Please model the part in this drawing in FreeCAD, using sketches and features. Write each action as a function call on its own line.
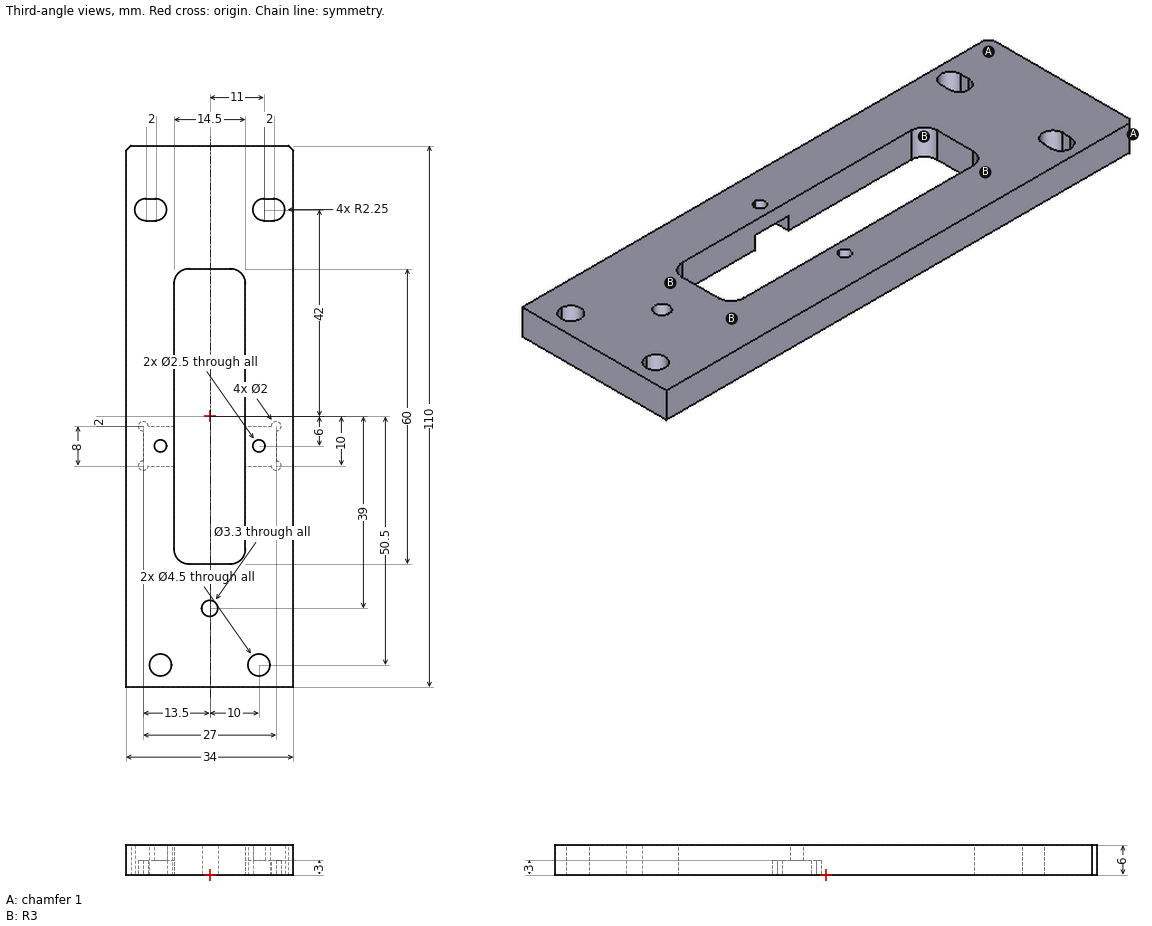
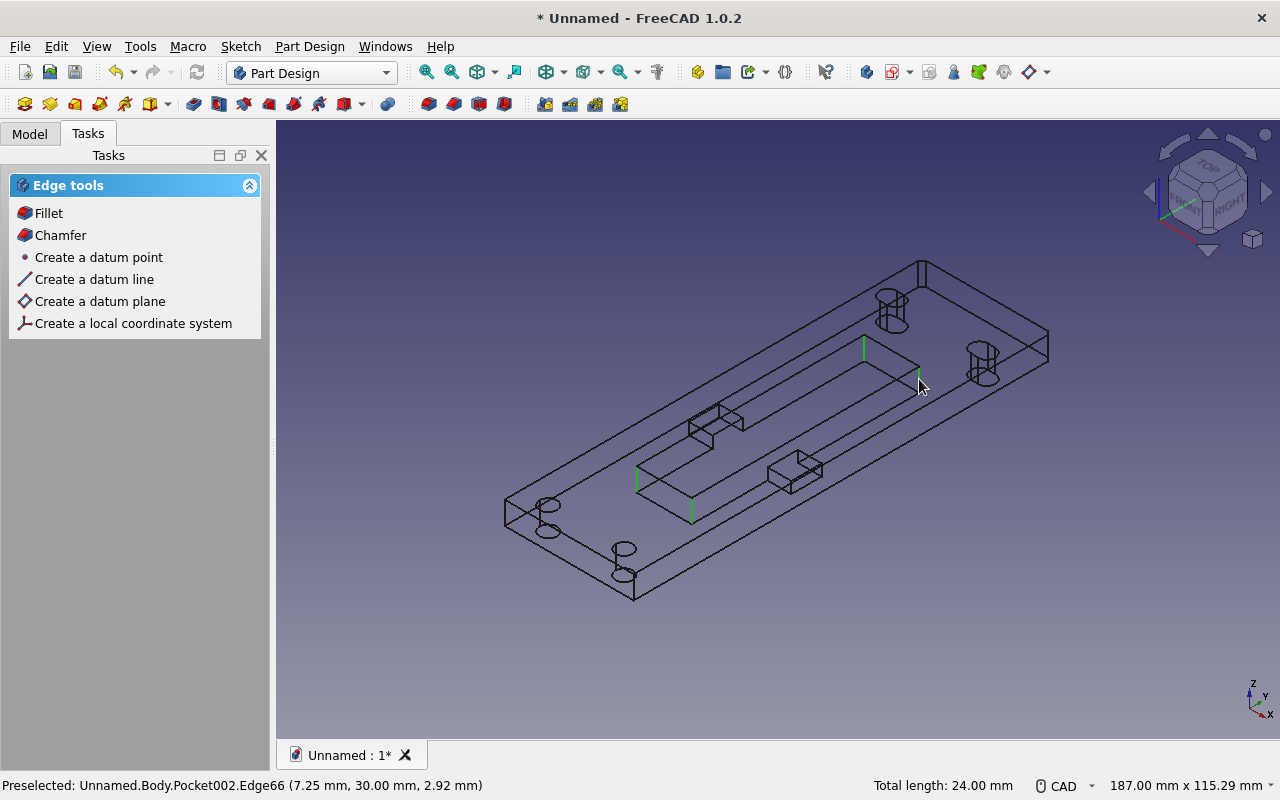
key(v)
key(1)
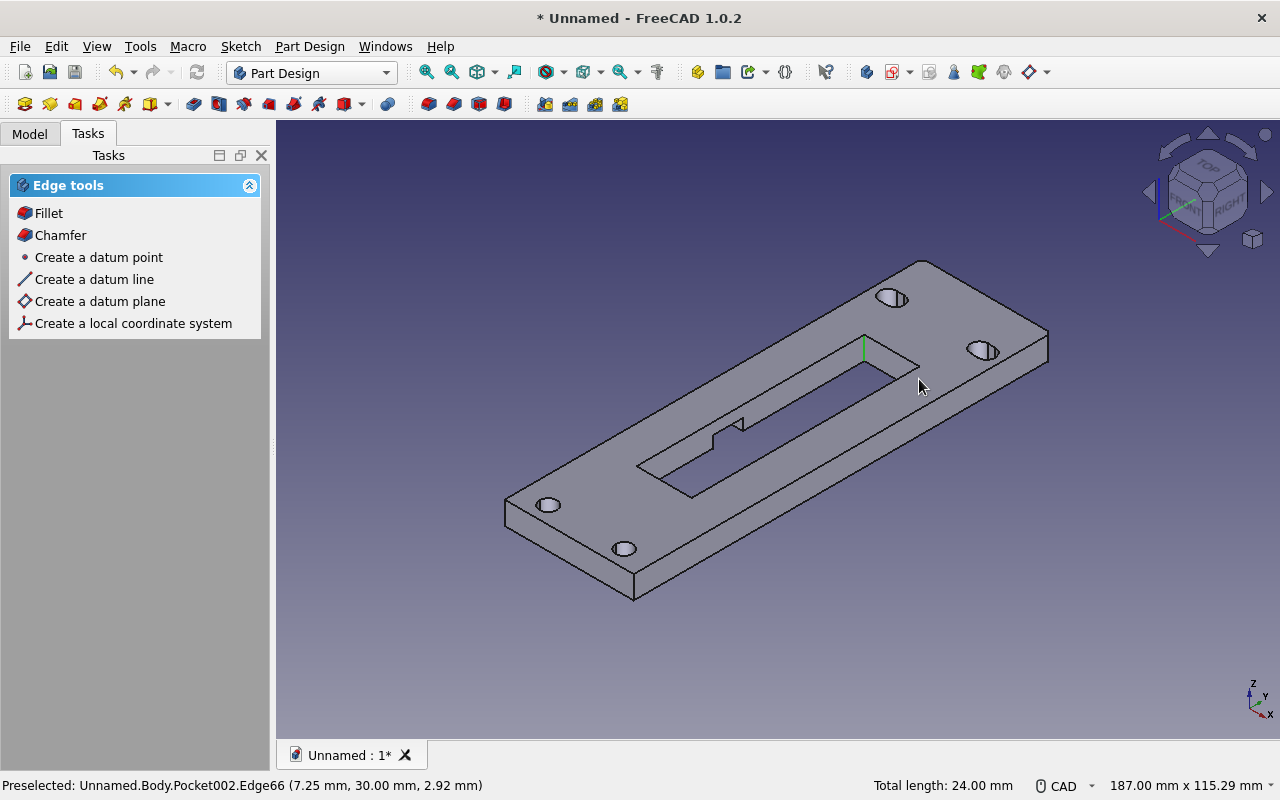
click(429, 104)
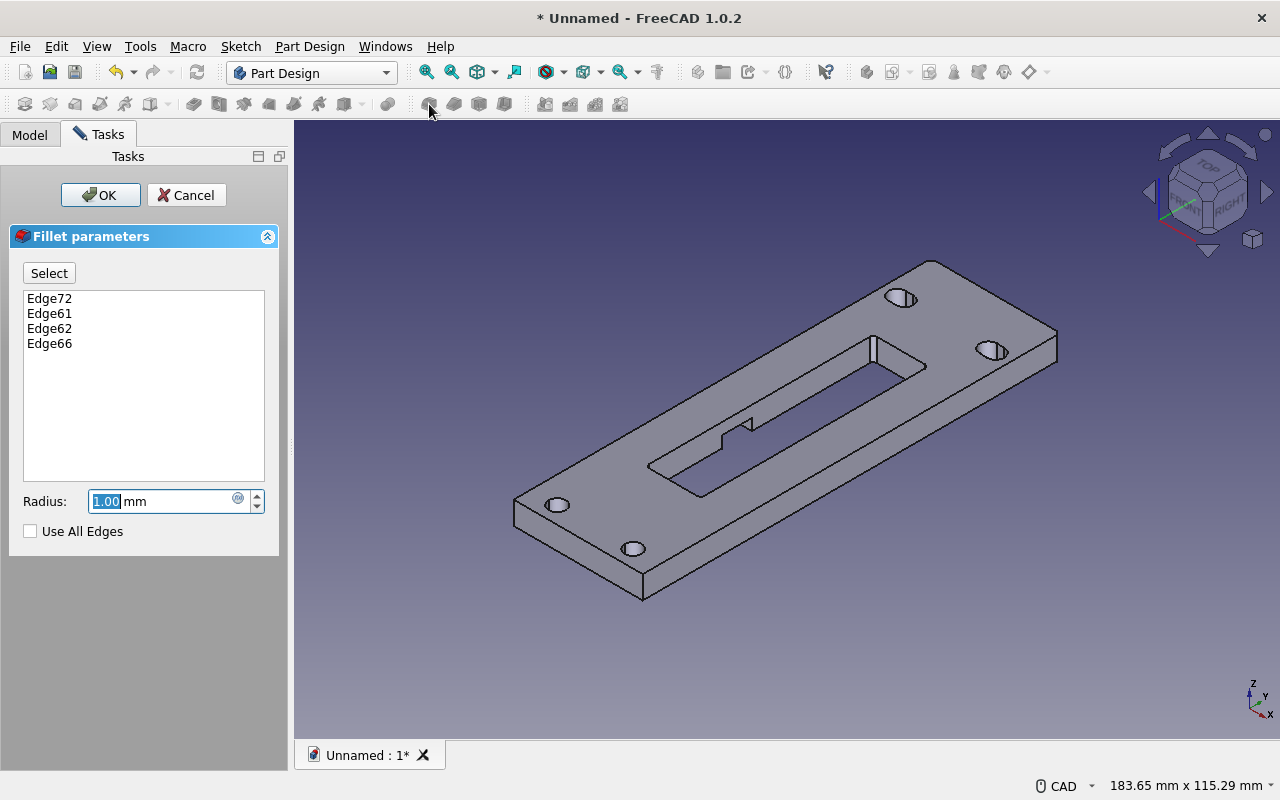
text(3)
key(Tab)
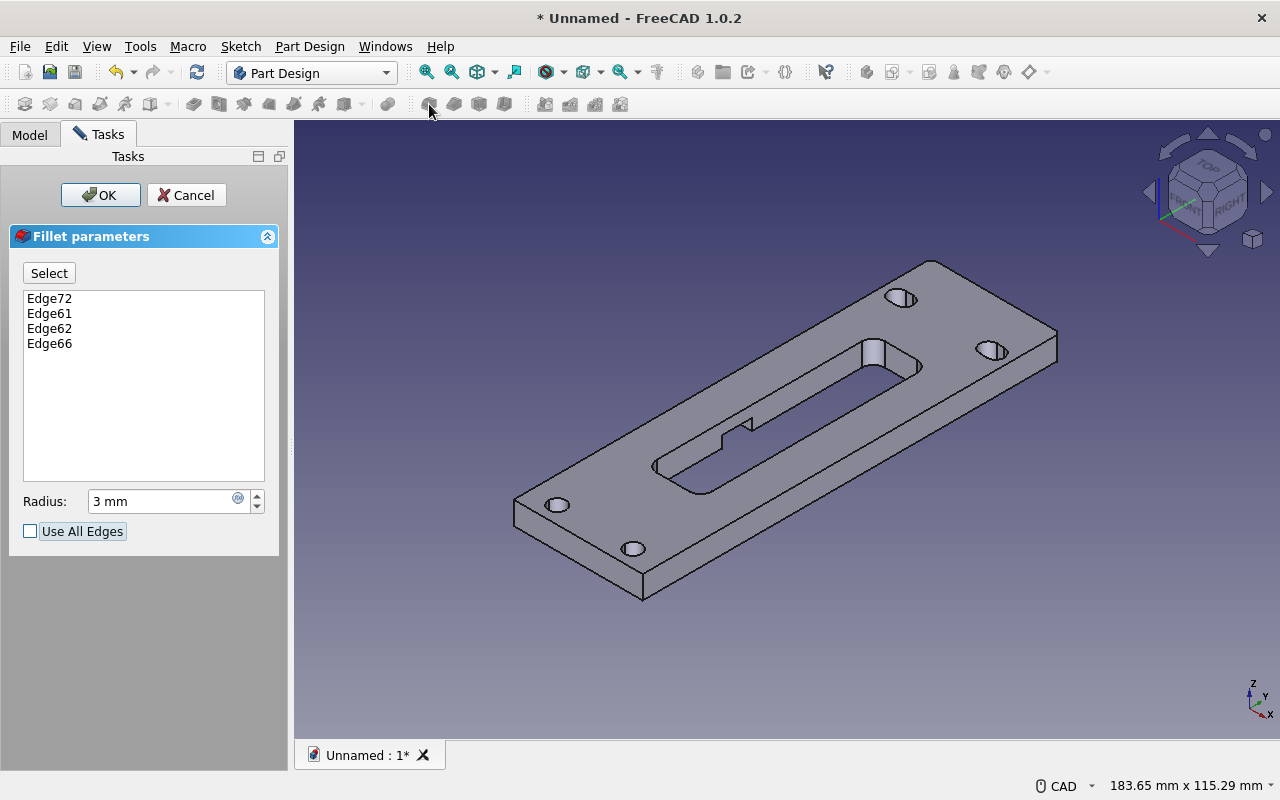
click(101, 195)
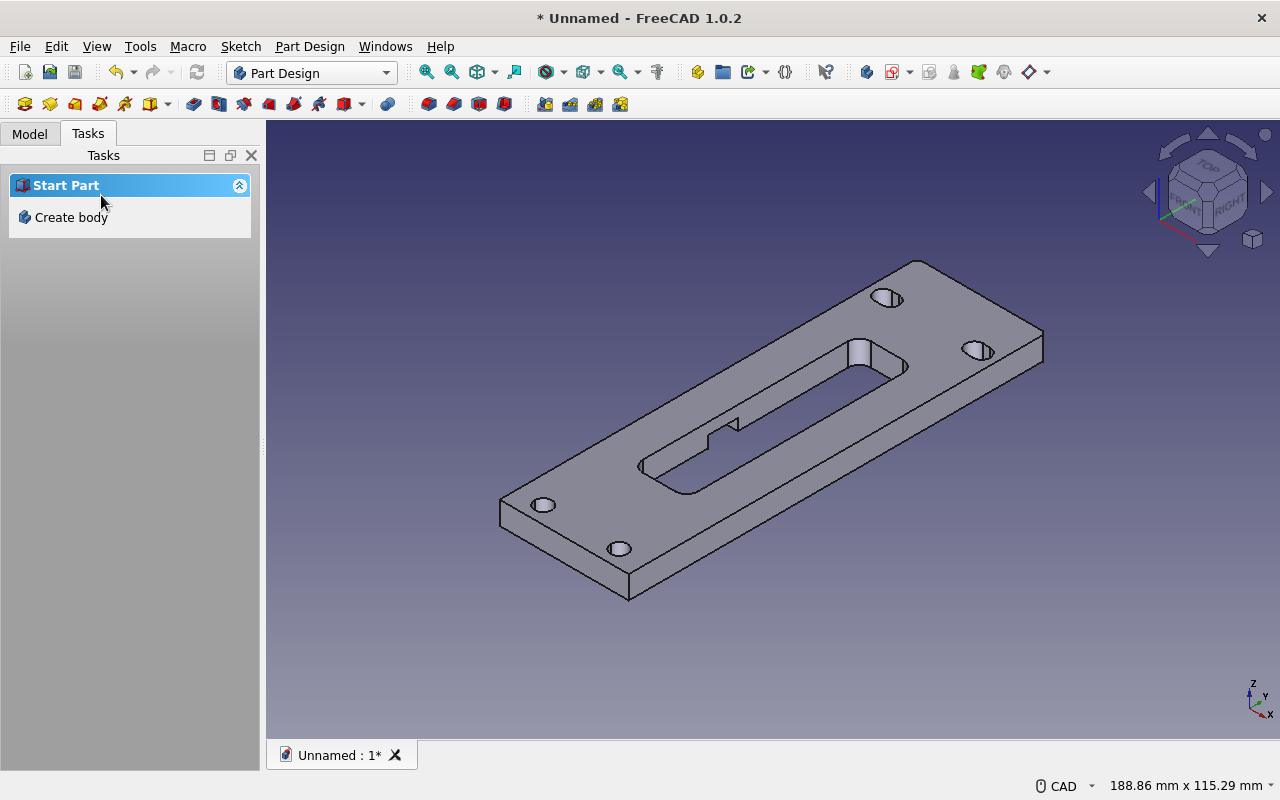
key(5)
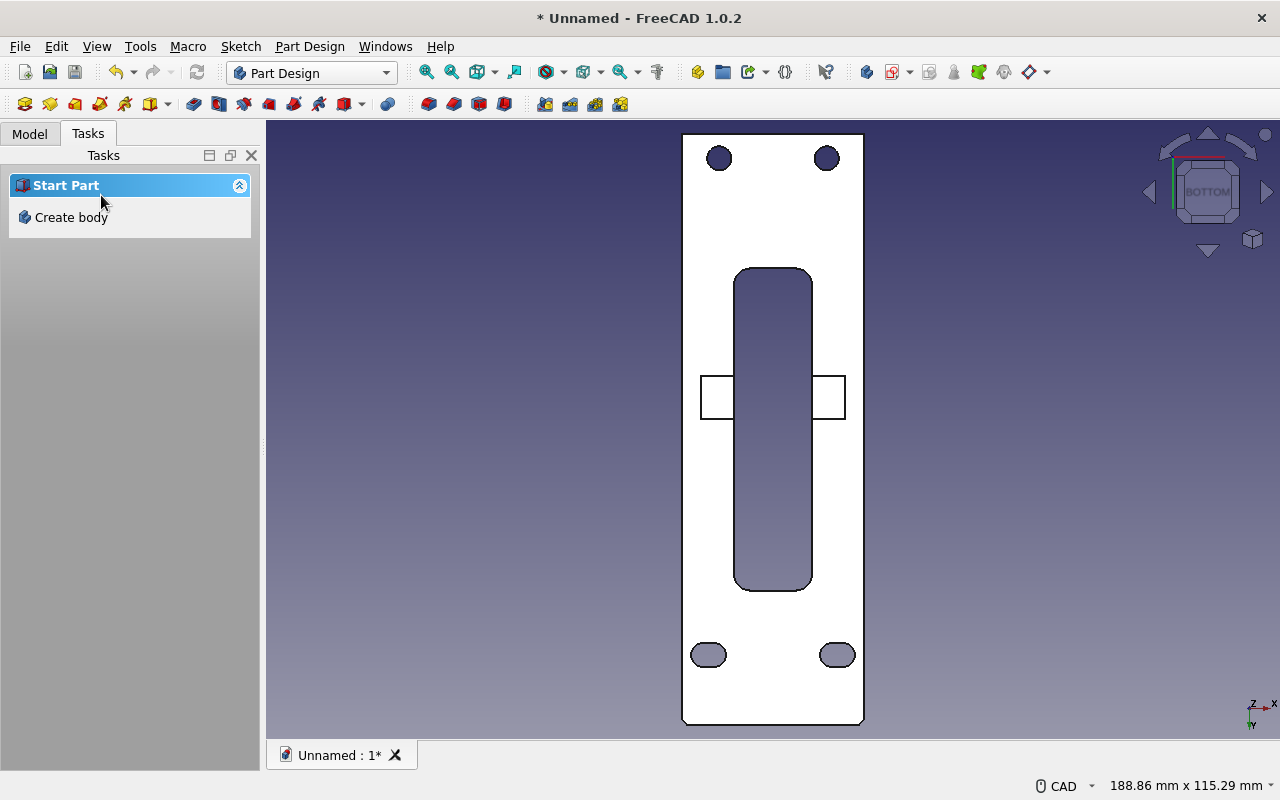
click(773, 682)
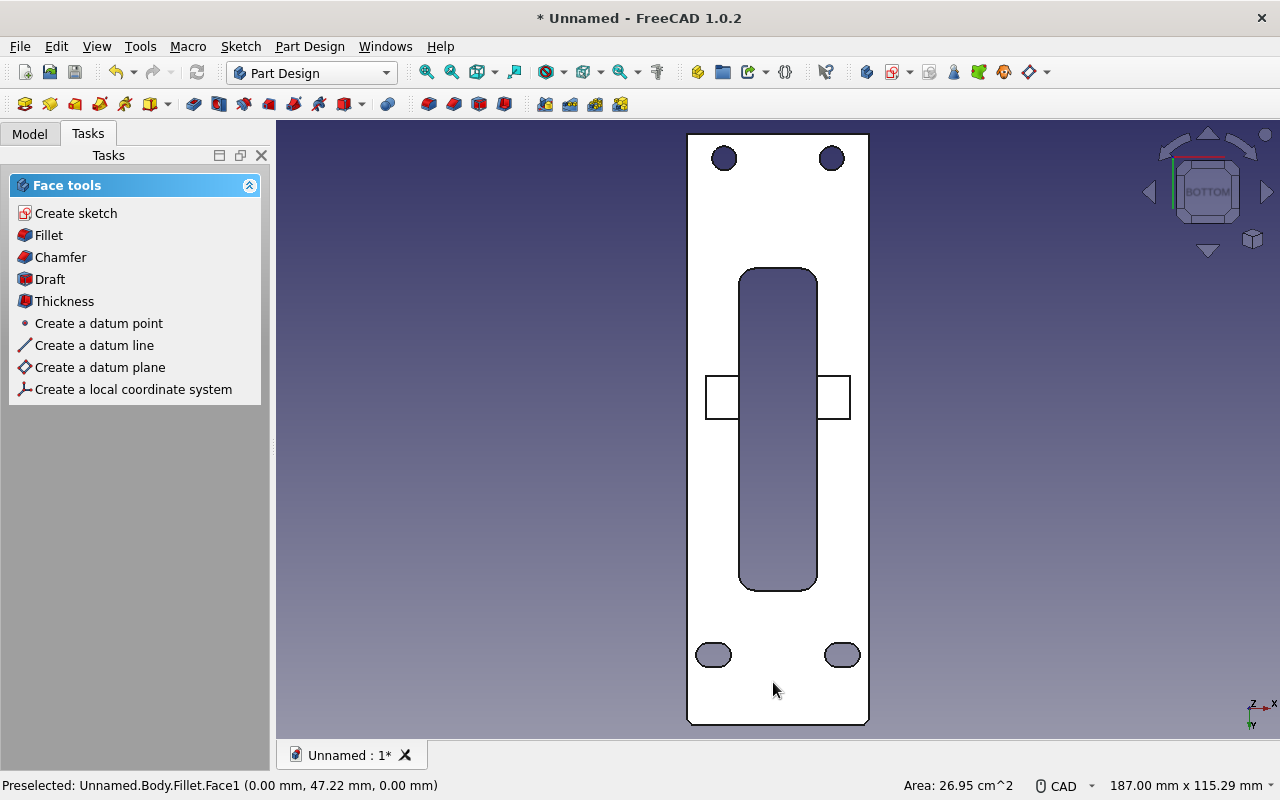
click(892, 72)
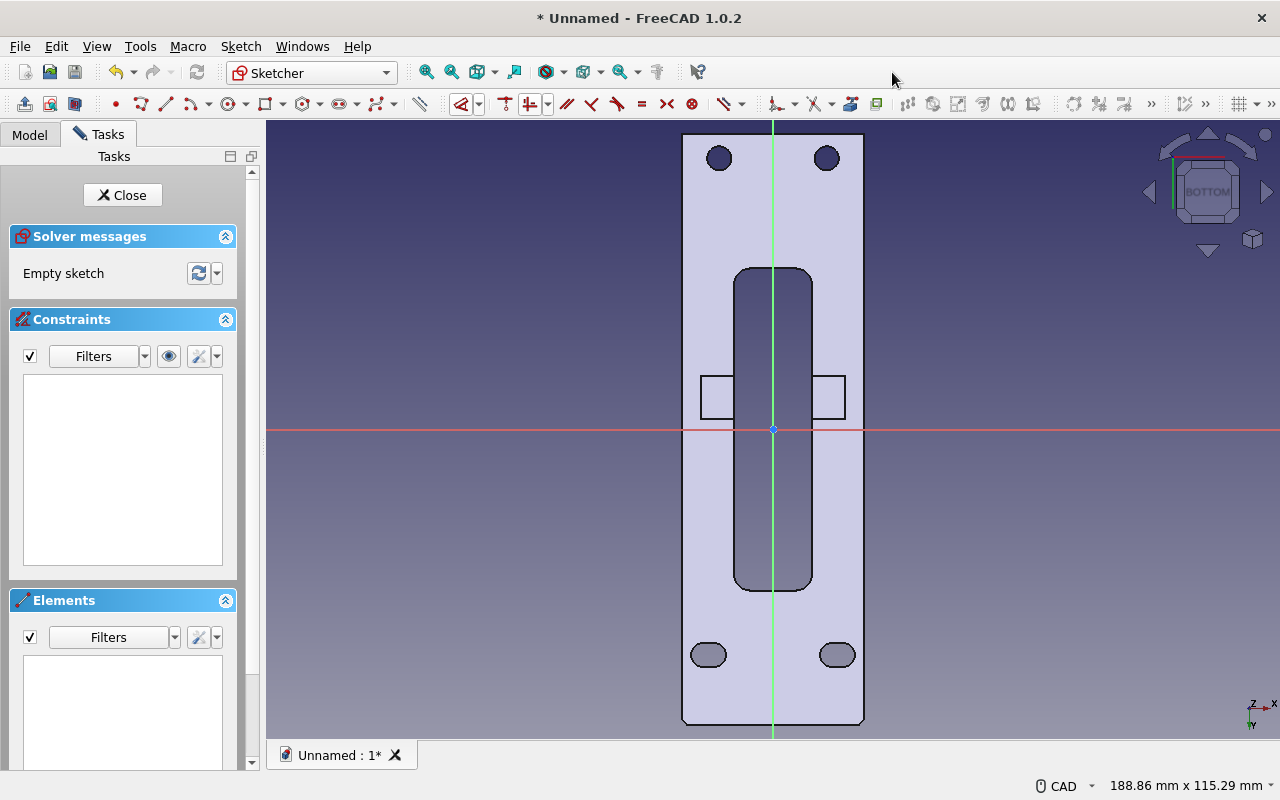
scroll(795, 390, up, 7)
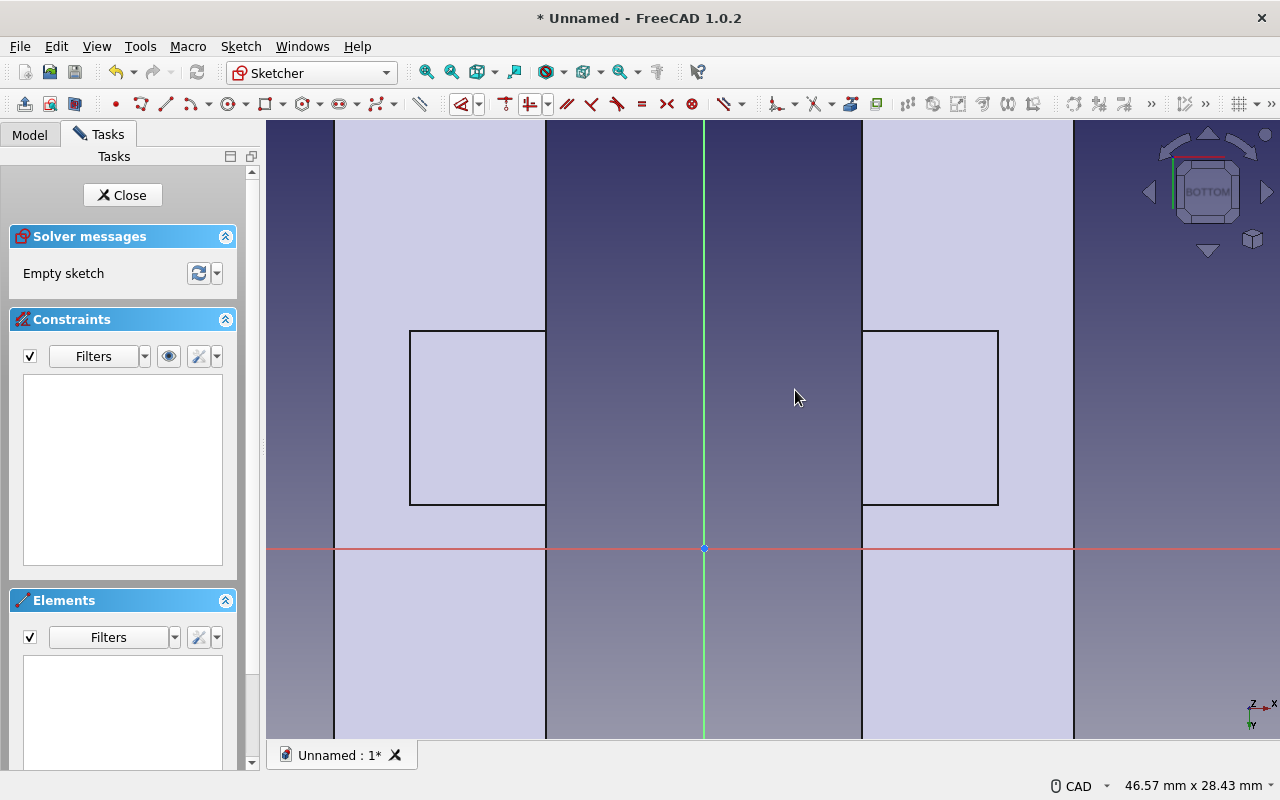
key(g)
key(c)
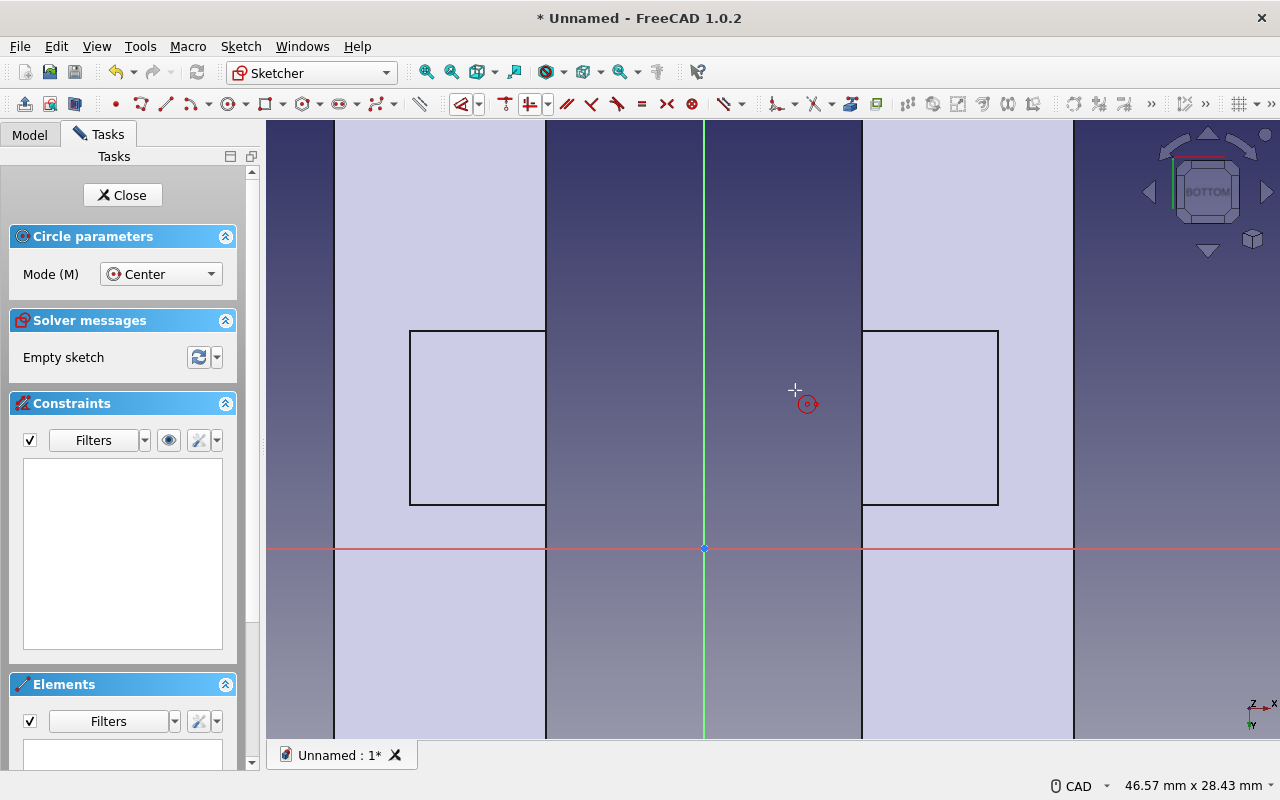
click(998, 505)
click(1014, 490)